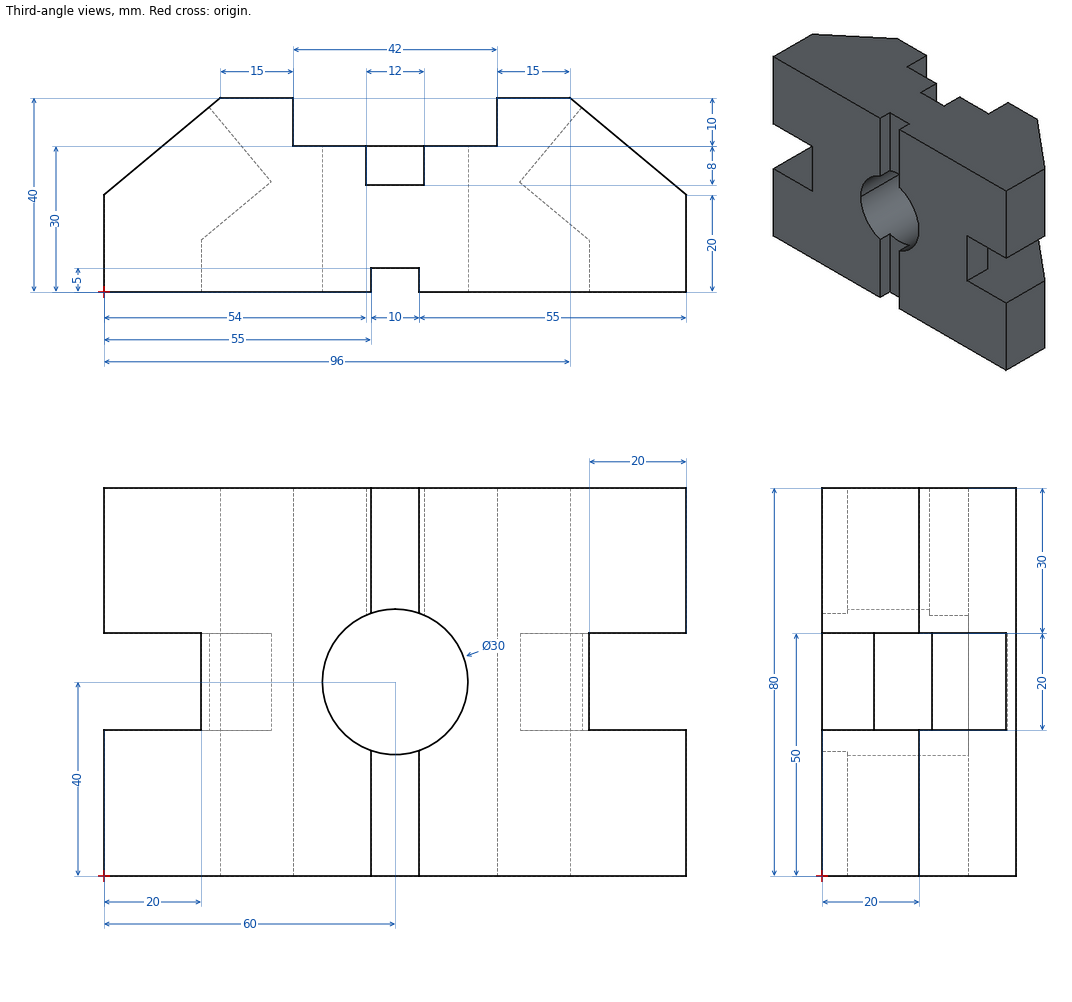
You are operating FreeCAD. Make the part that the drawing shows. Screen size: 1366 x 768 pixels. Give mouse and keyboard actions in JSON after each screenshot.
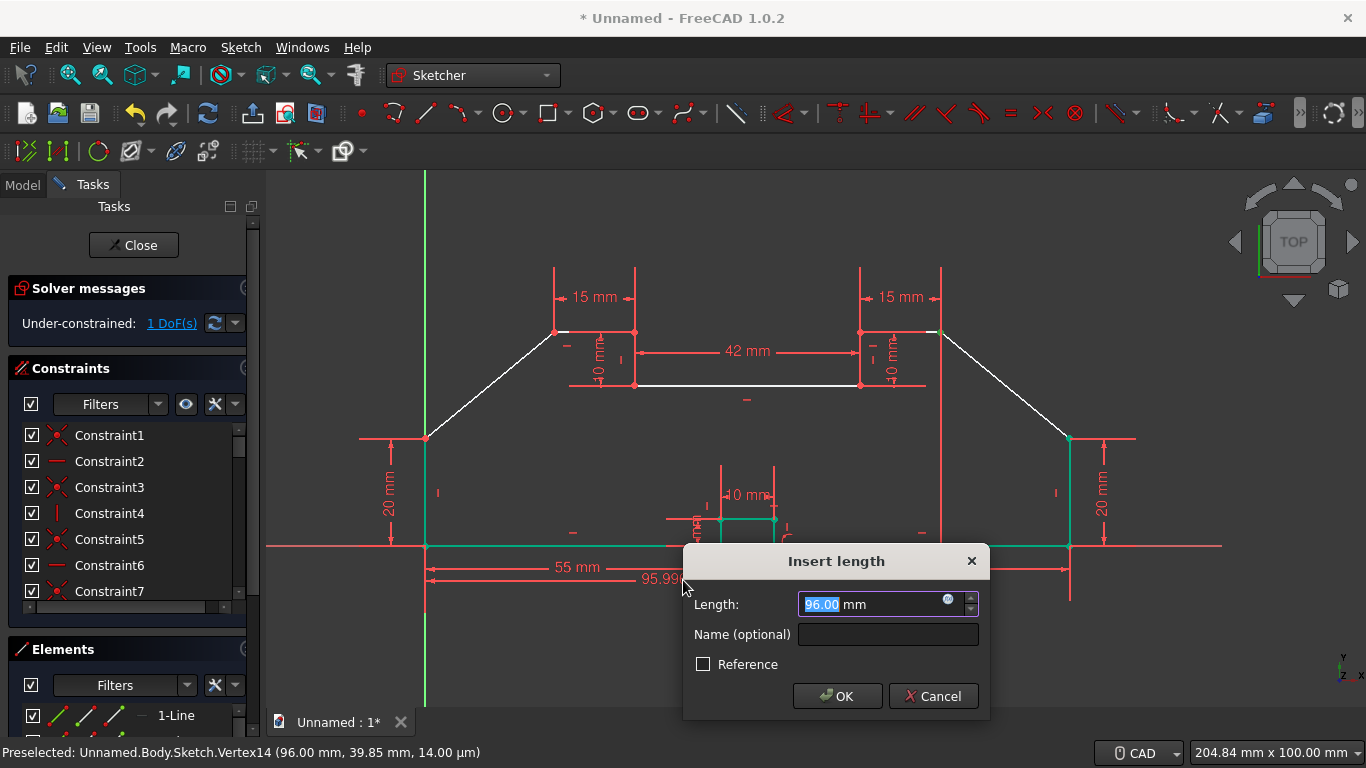
{"action": "type", "text": "96"}
{"action": "key", "text": "Return"}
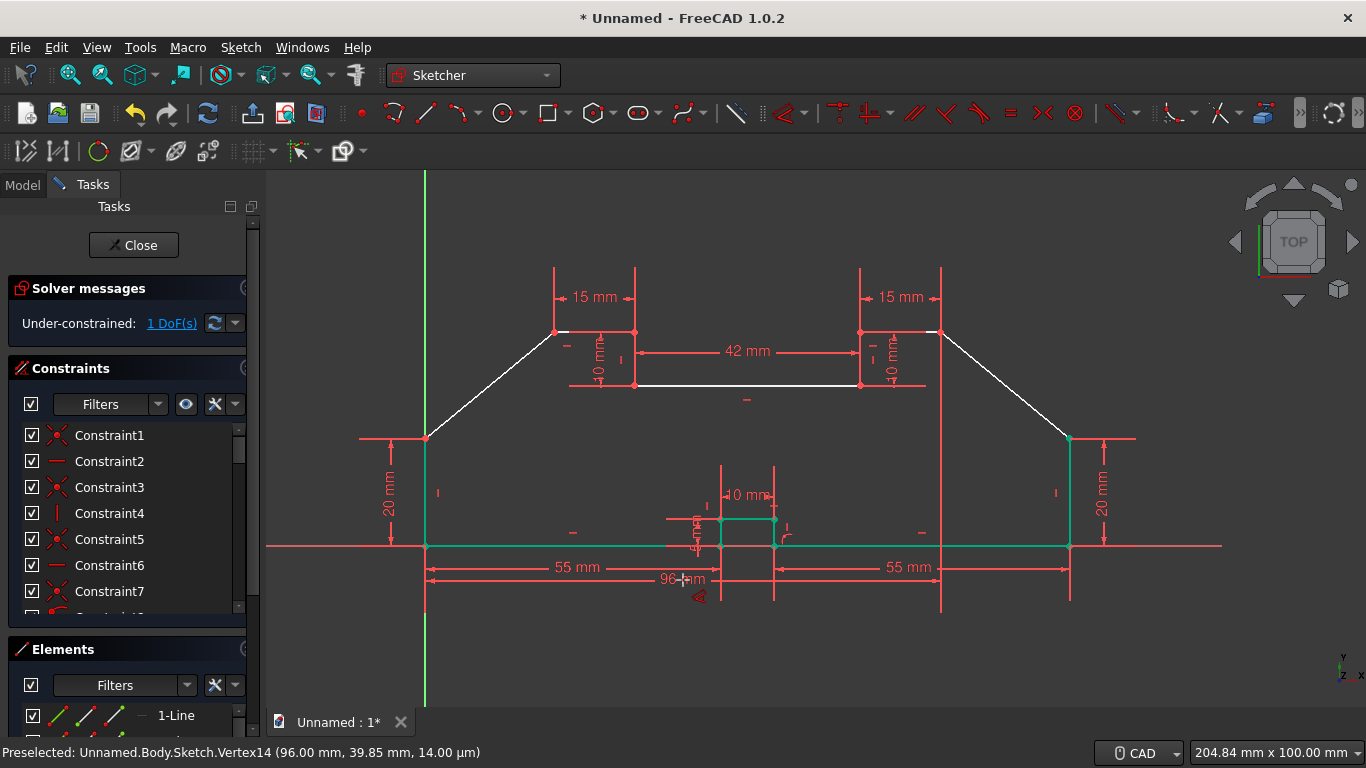
{"action": "left_click", "coordinate": [941, 332]}
{"action": "left_click", "coordinate": [391, 439]}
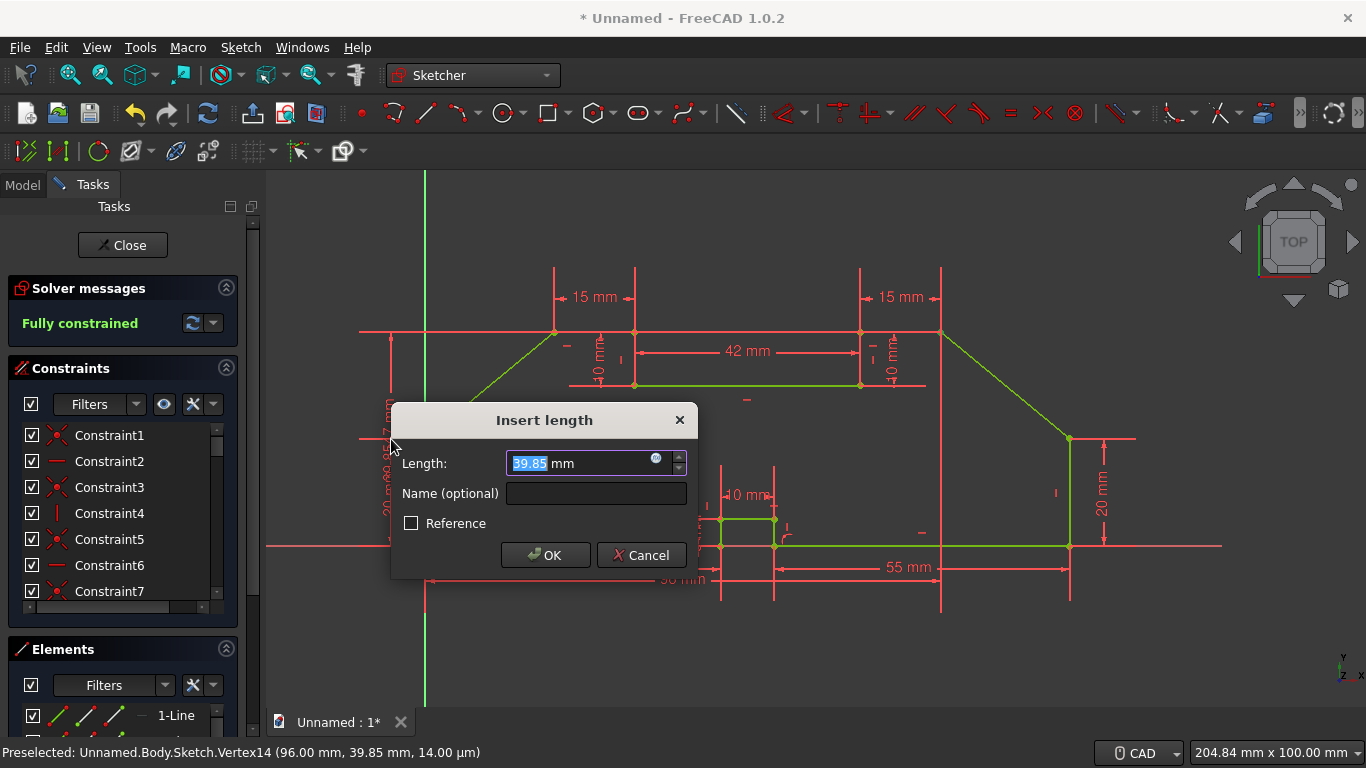
{"action": "type", "text": "40"}
{"action": "key", "text": "Return"}
{"action": "key", "text": "Escape"}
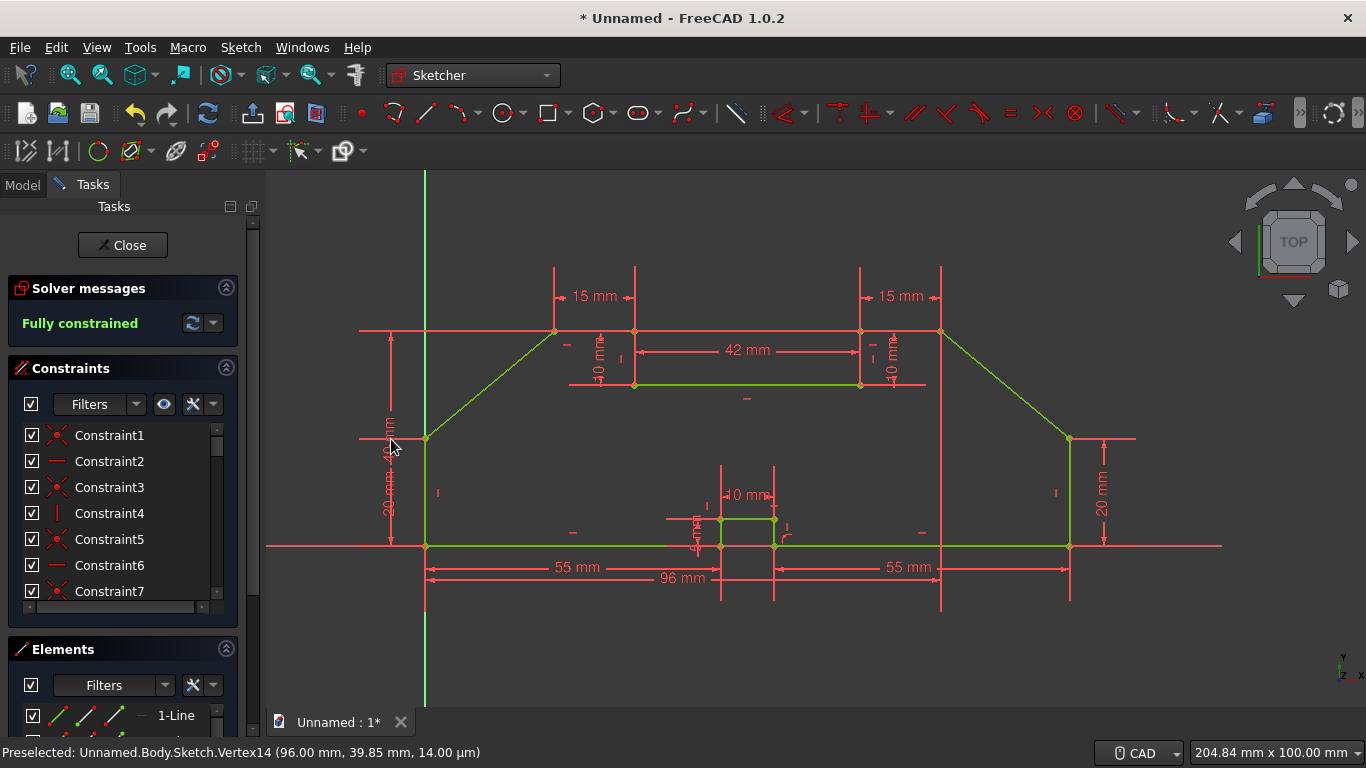
{"action": "left_click", "coordinate": [123, 245]}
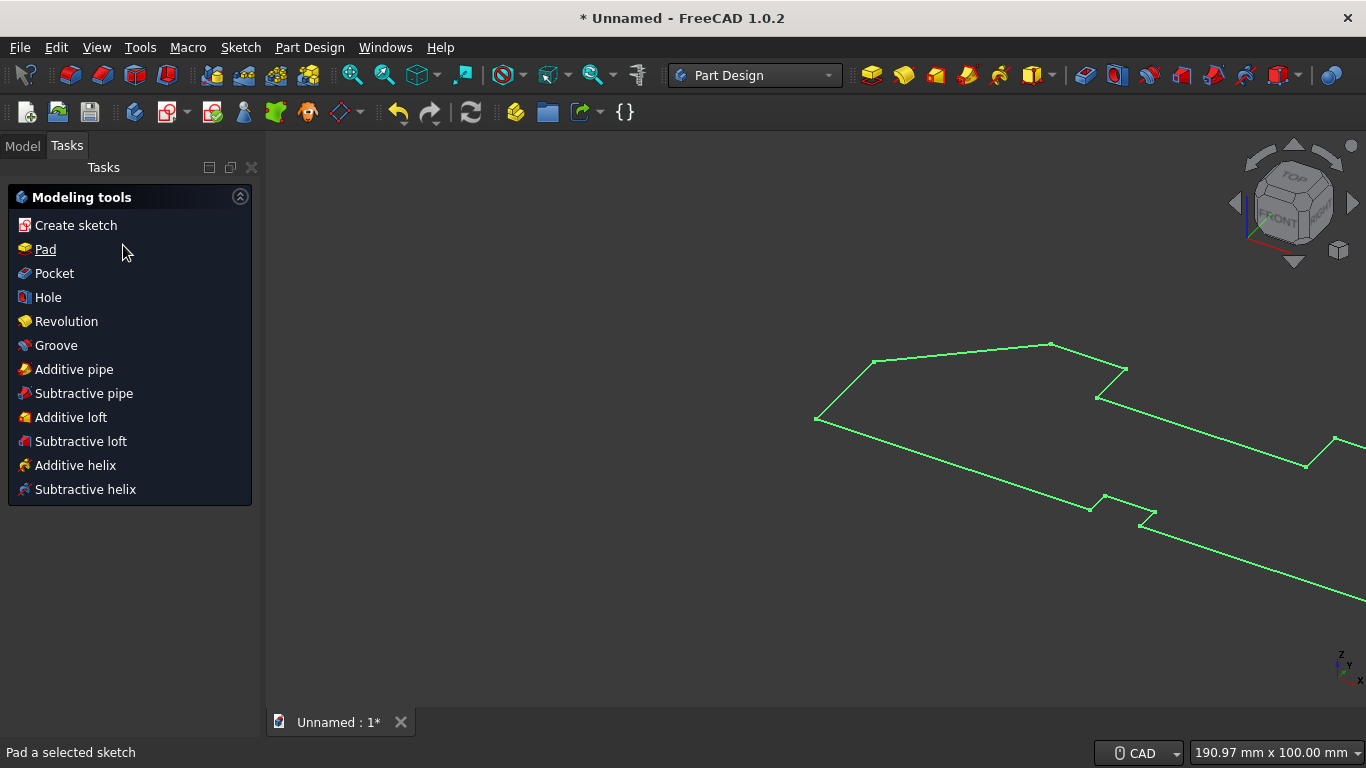
{"action": "left_click", "coordinate": [872, 76]}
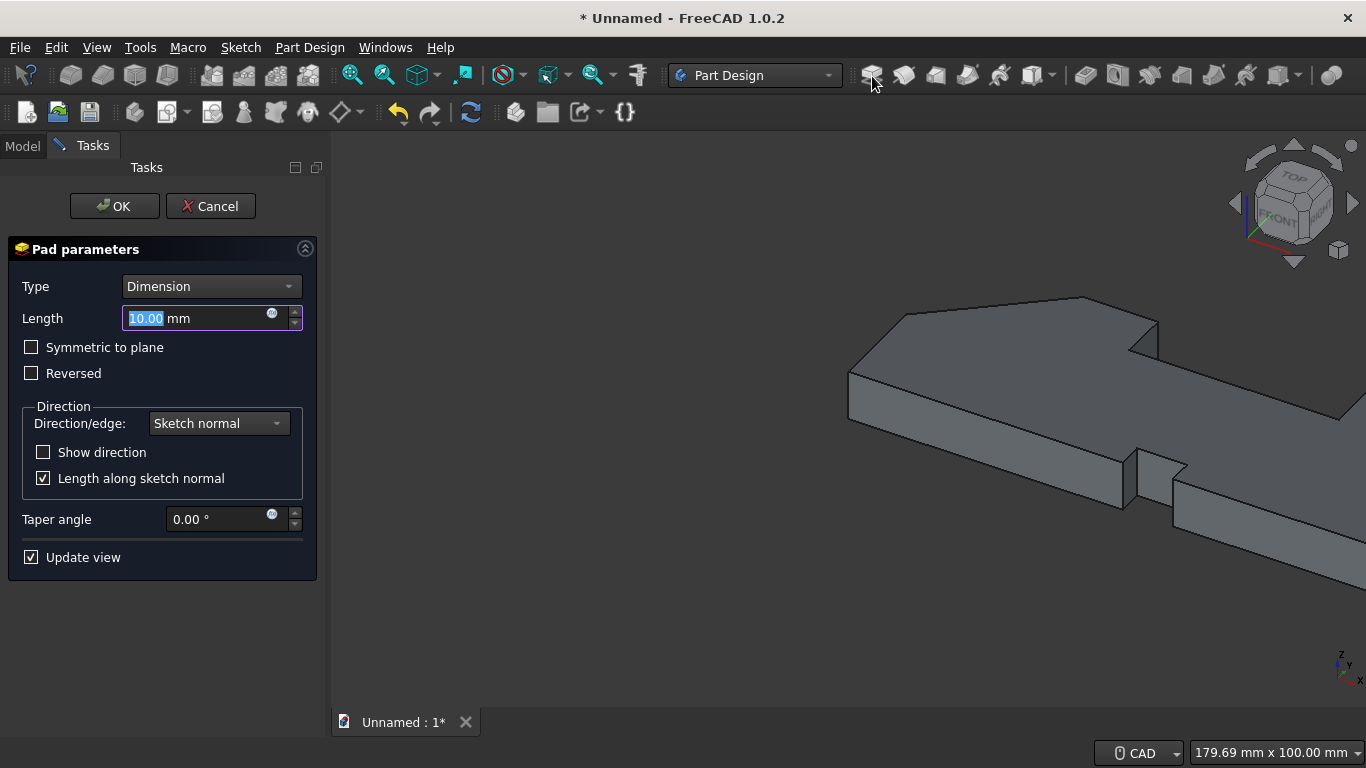
{"action": "type", "text": "80"}
{"action": "key", "text": "Tab"}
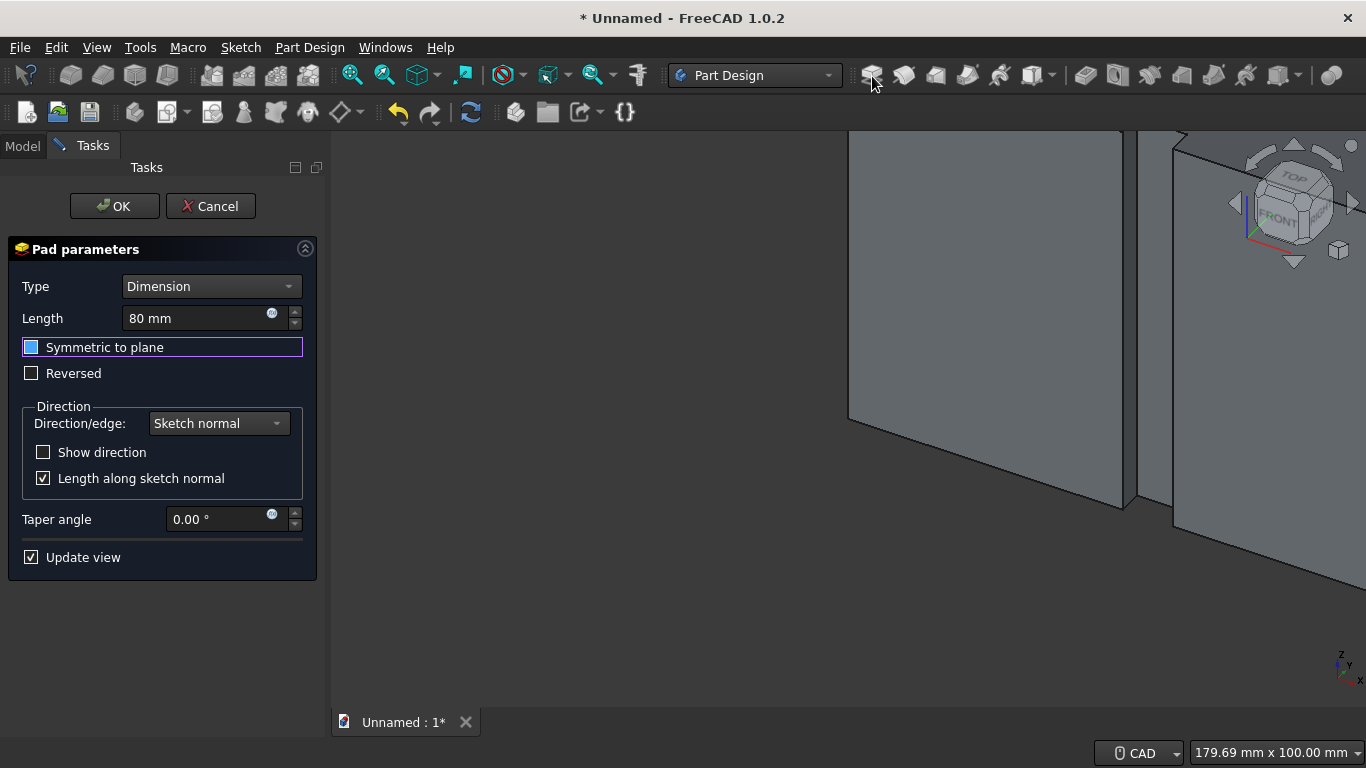
{"action": "left_click", "coordinate": [115, 206]}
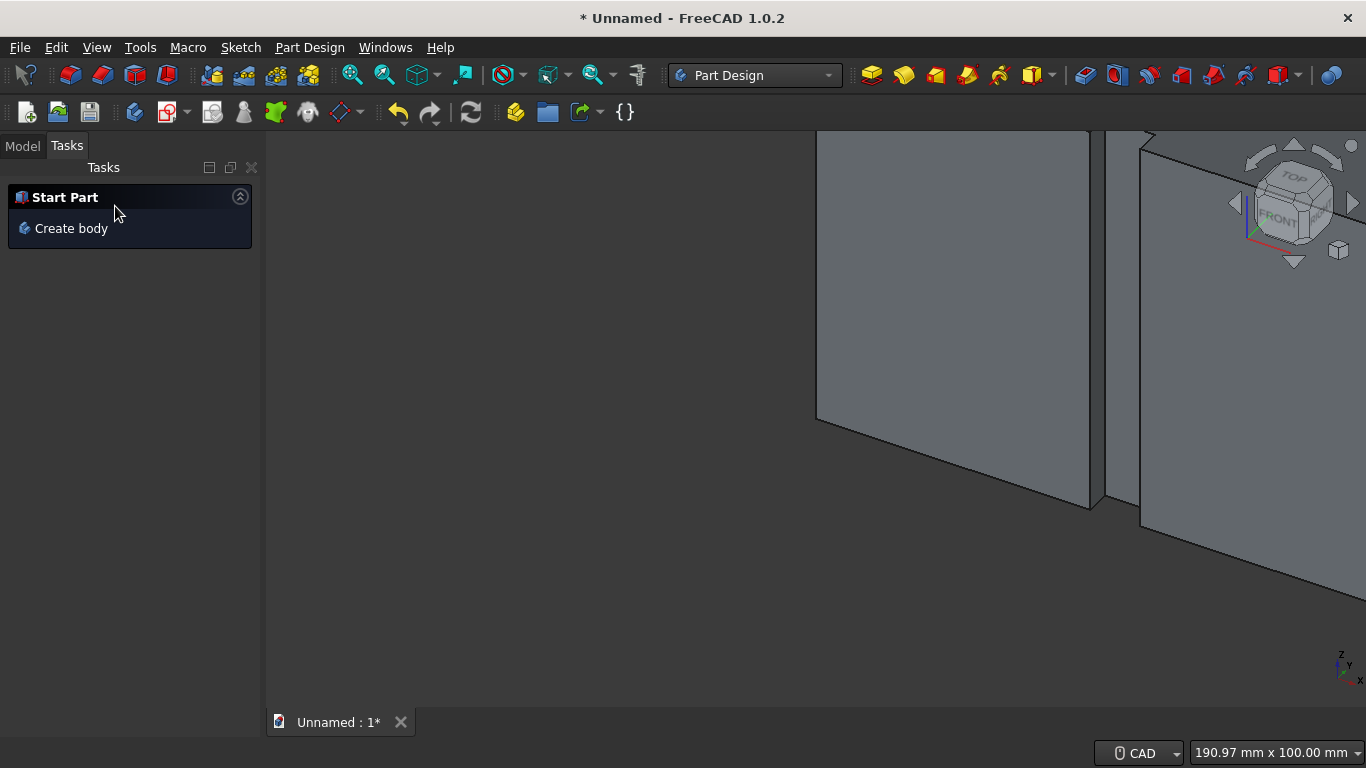
{"action": "key", "text": "v f"}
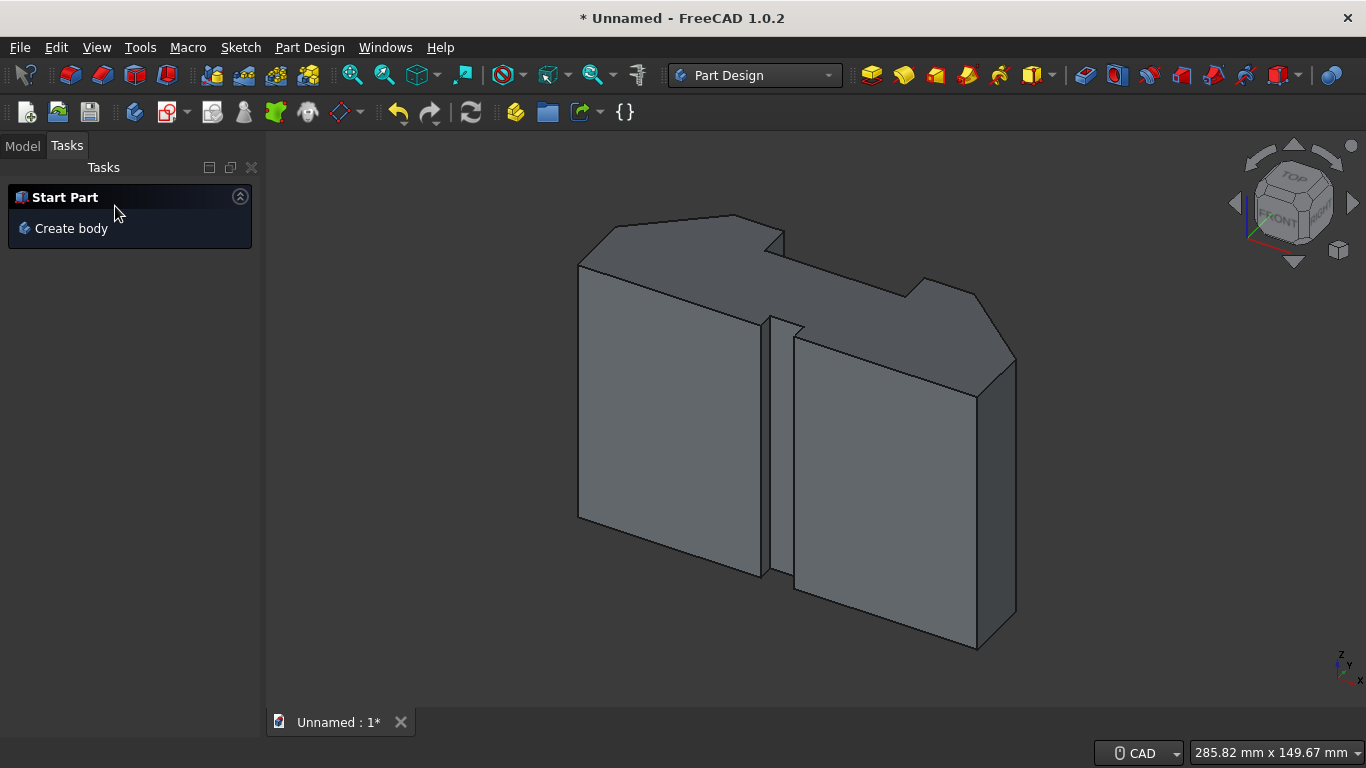
{"action": "key", "text": "4"}